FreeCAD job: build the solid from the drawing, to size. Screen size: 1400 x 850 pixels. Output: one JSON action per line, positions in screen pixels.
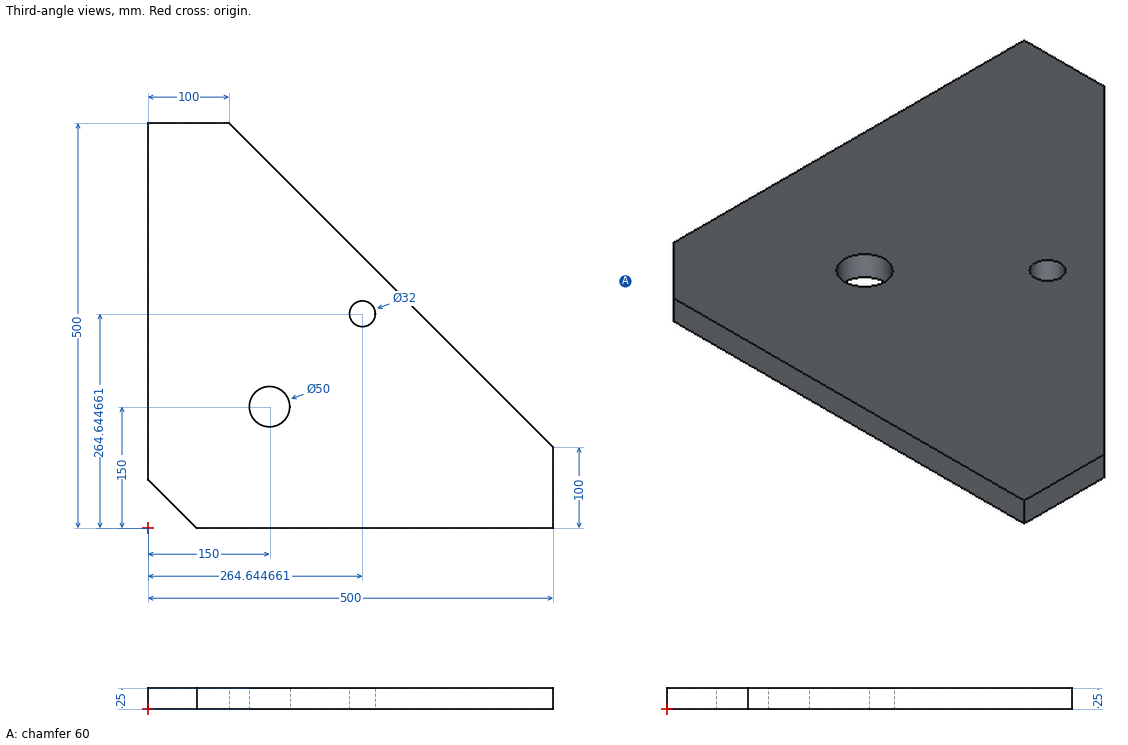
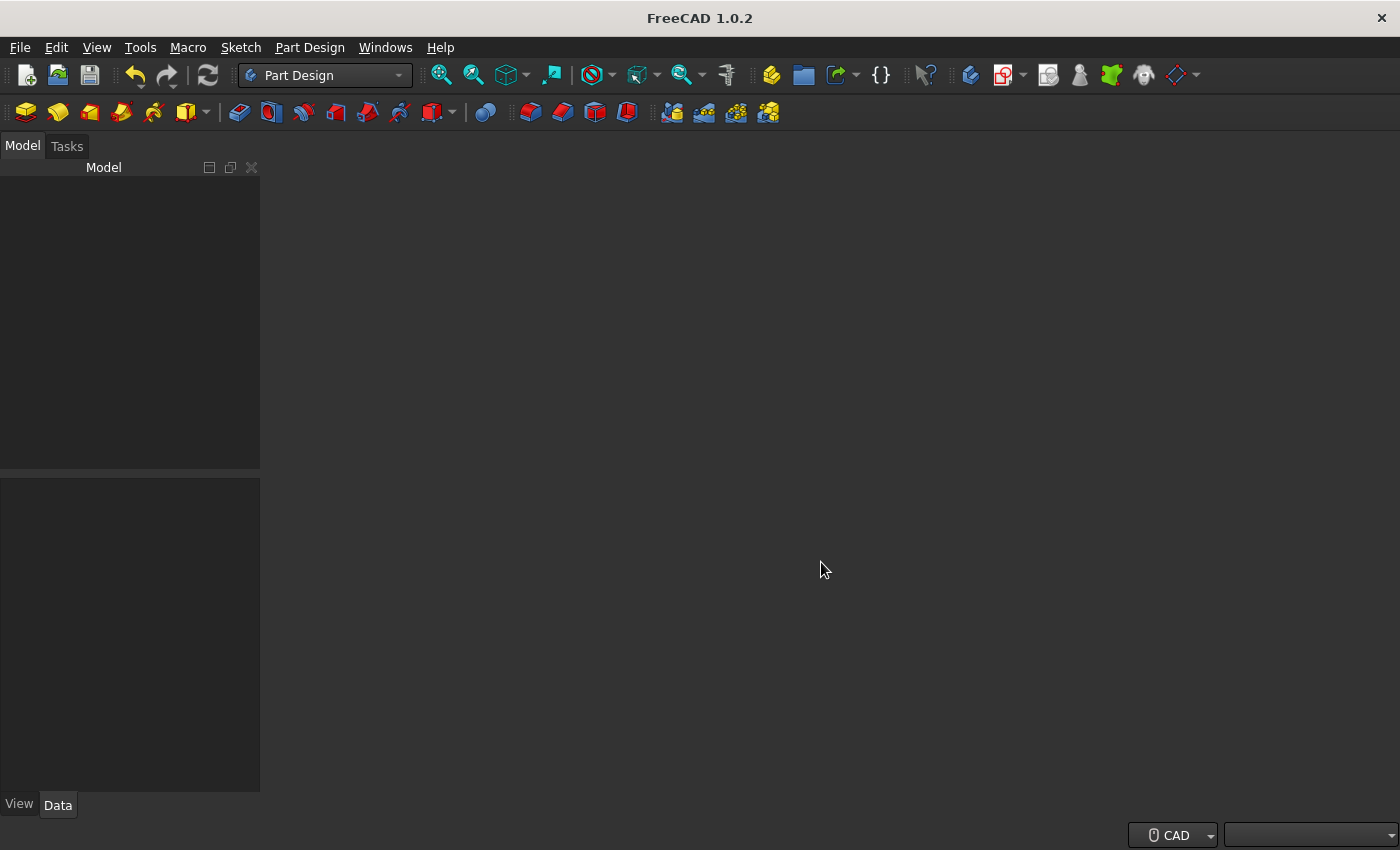
{"action": "left_click", "coordinate": [26, 76]}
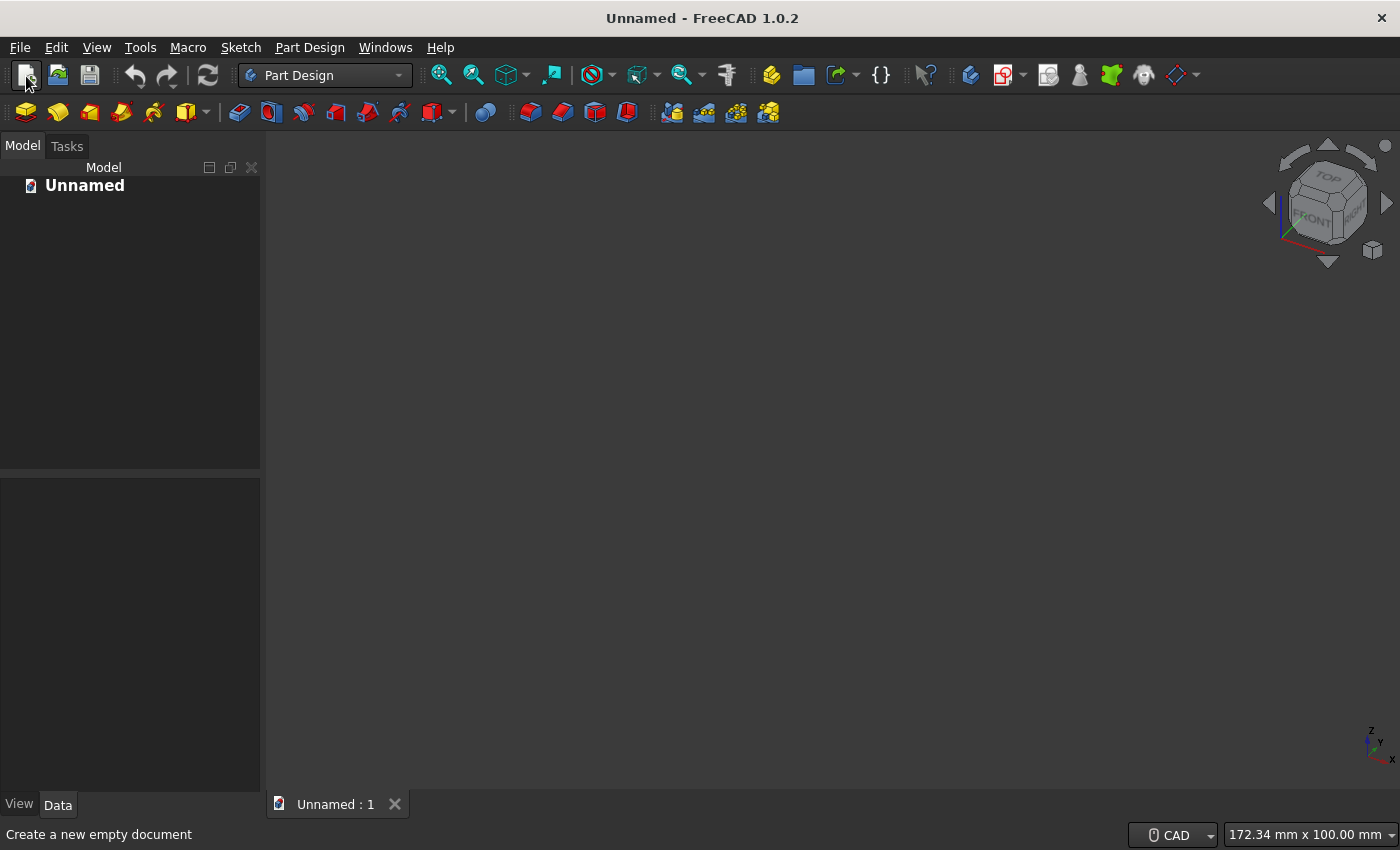
{"action": "left_click", "coordinate": [1004, 76]}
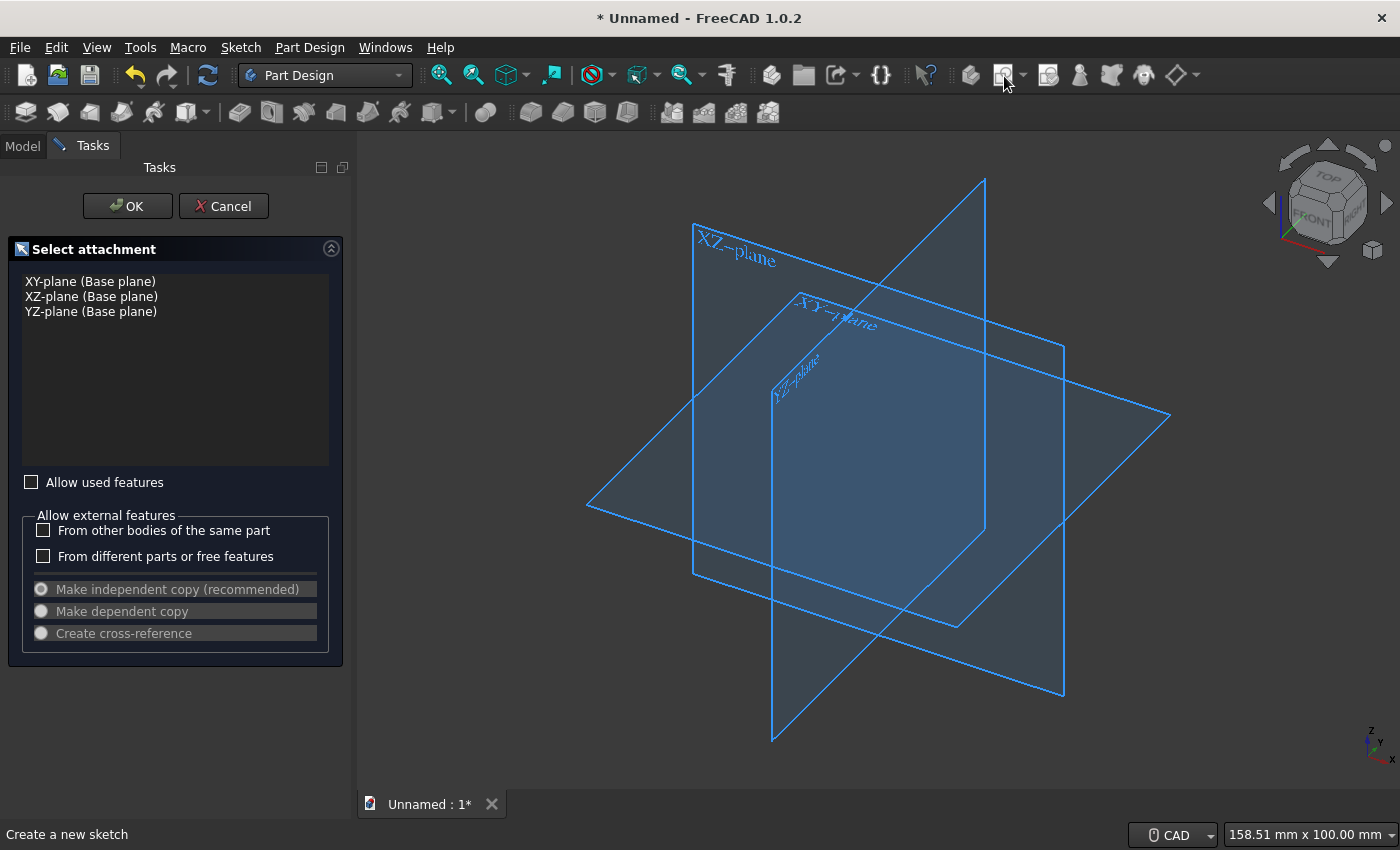
{"action": "left_click", "coordinate": [82, 282]}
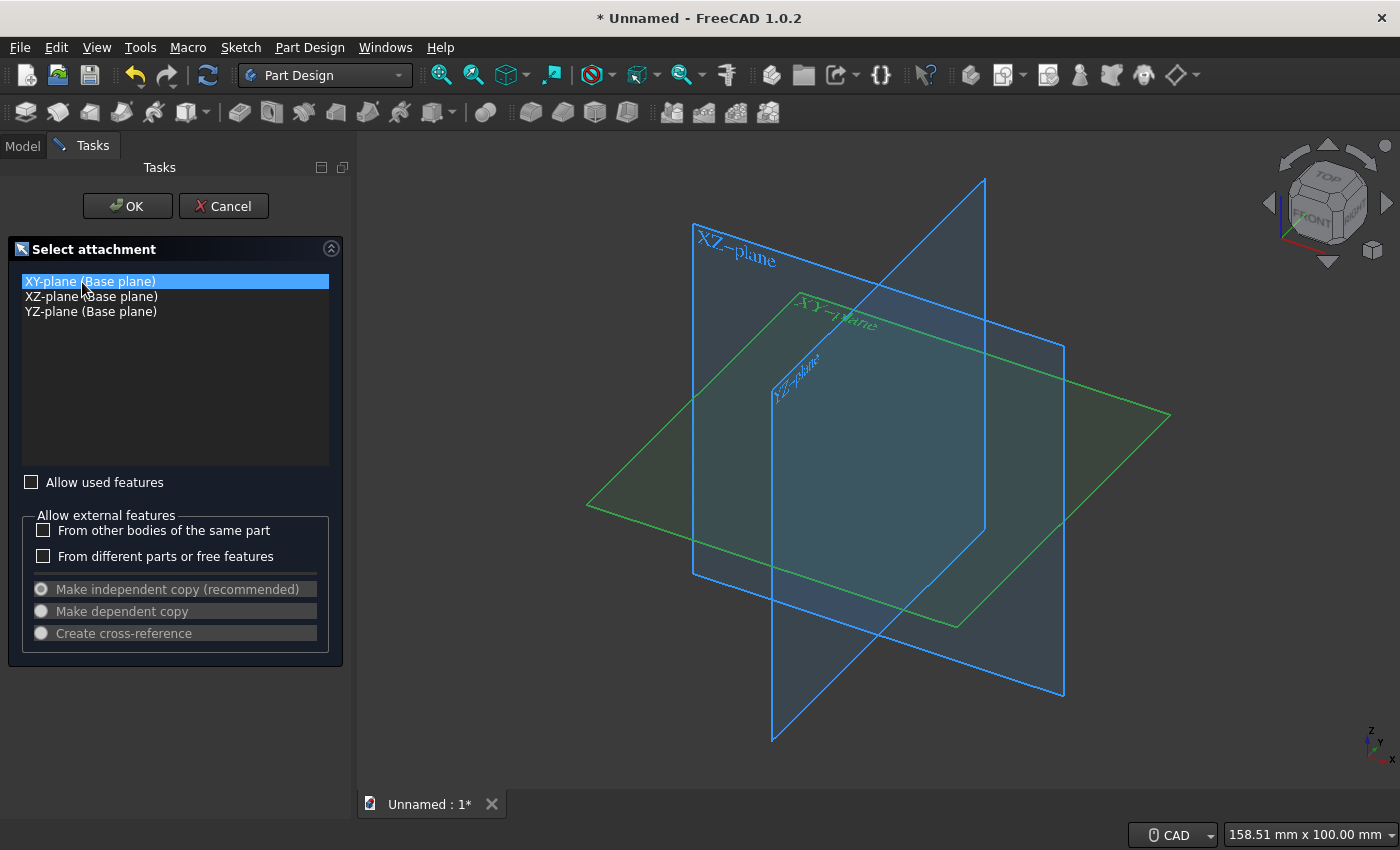
{"action": "left_click", "coordinate": [128, 206]}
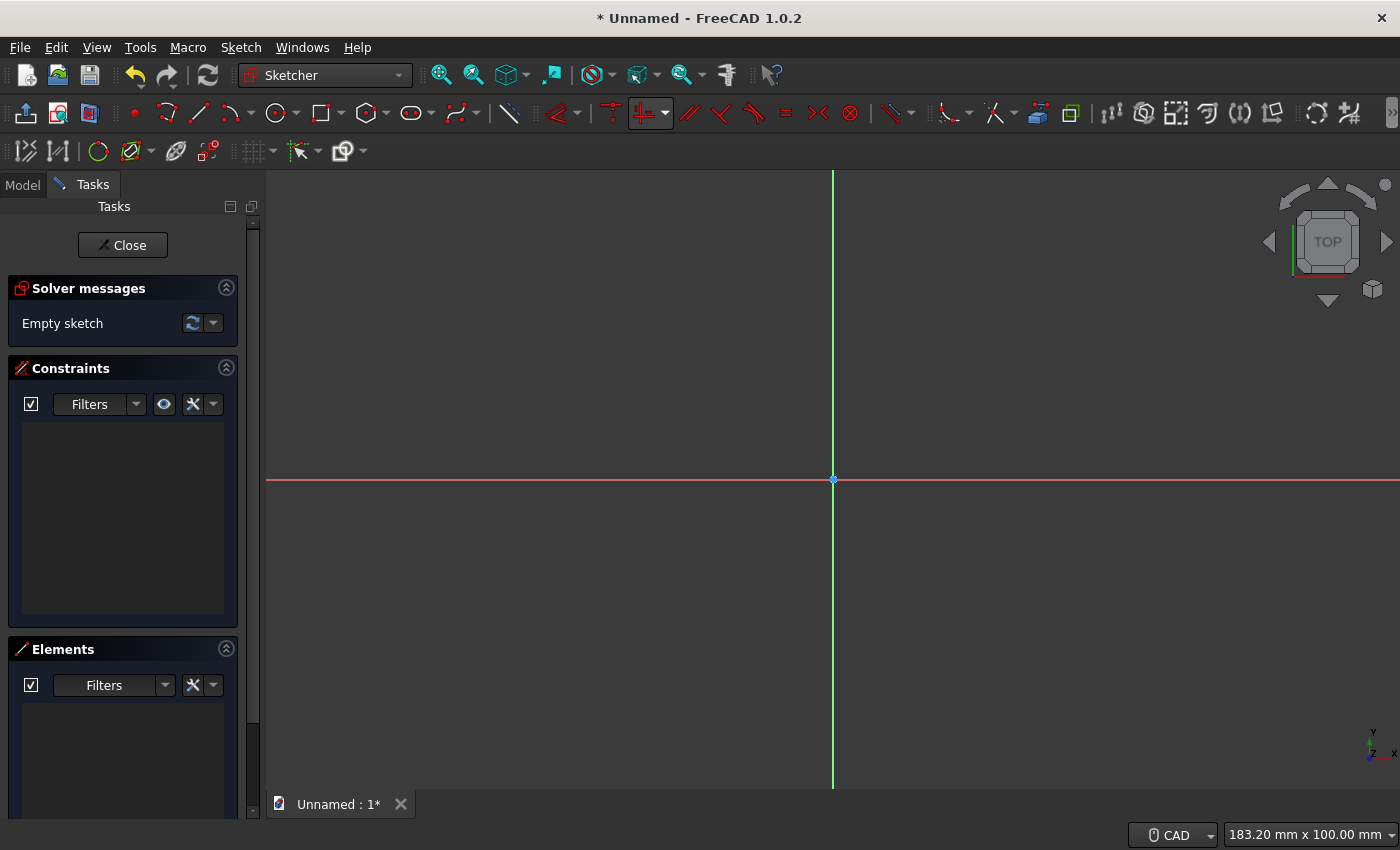
{"action": "scroll", "coordinate": [512, 722], "scroll_direction": "down", "scroll_amount": 10}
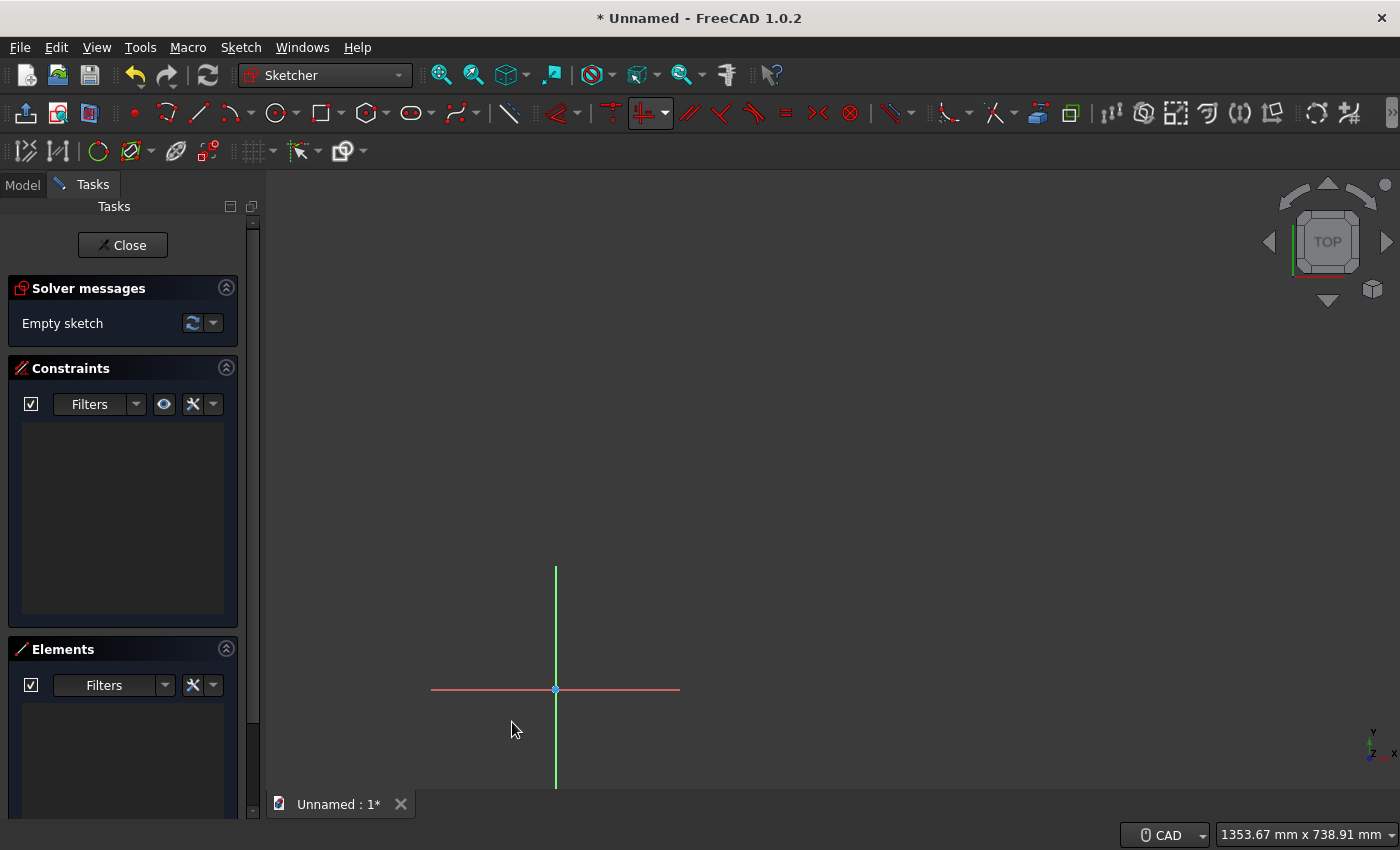
{"action": "left_click", "coordinate": [168, 114]}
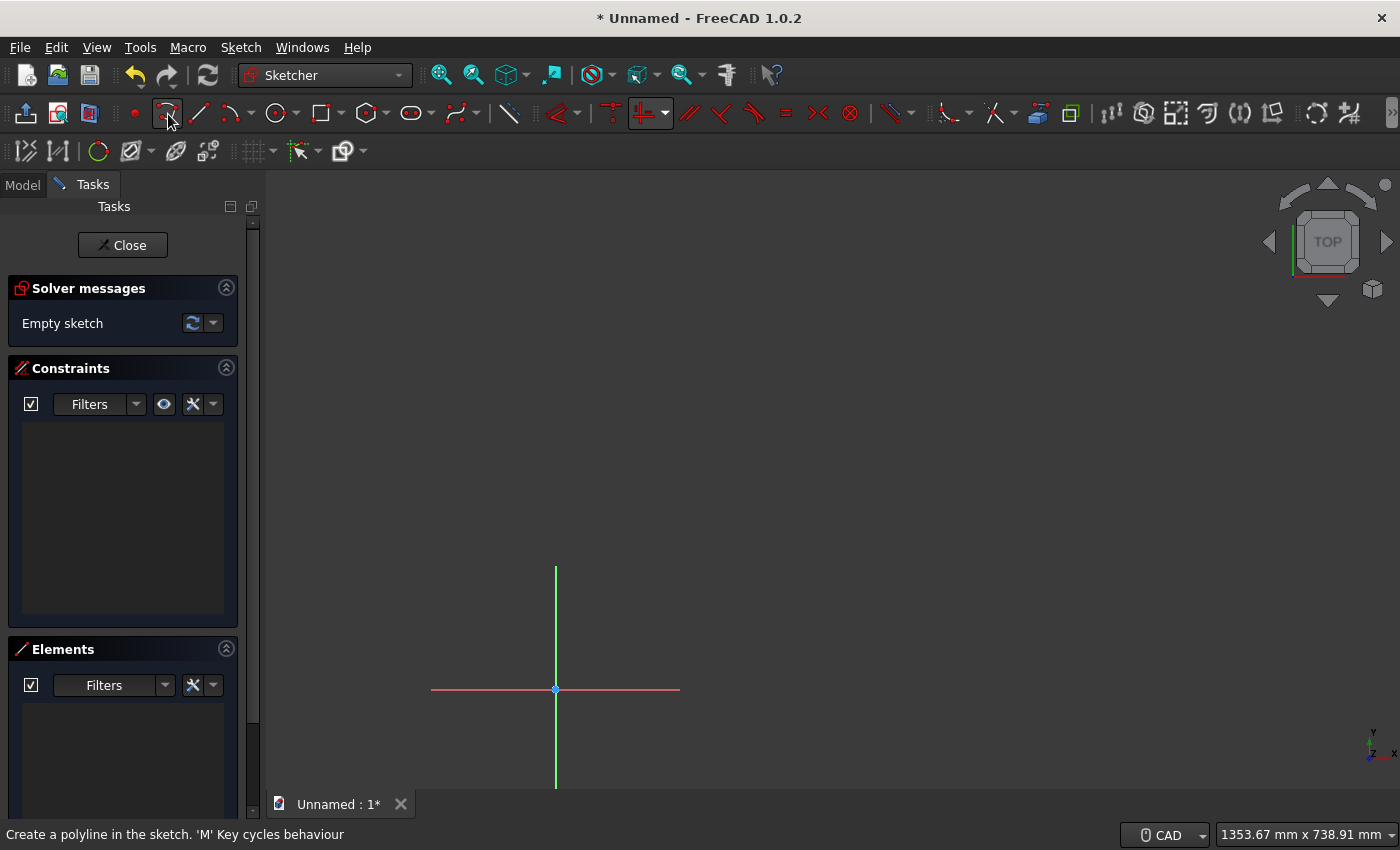
{"action": "left_click", "coordinate": [556, 690]}
{"action": "left_click", "coordinate": [974, 681]}
{"action": "left_click", "coordinate": [974, 606]}
{"action": "left_click", "coordinate": [639, 271]}
{"action": "left_click", "coordinate": [565, 271]}
{"action": "left_click", "coordinate": [556, 690]}
{"action": "key", "text": "Escape"}
{"action": "key", "text": "Escape"}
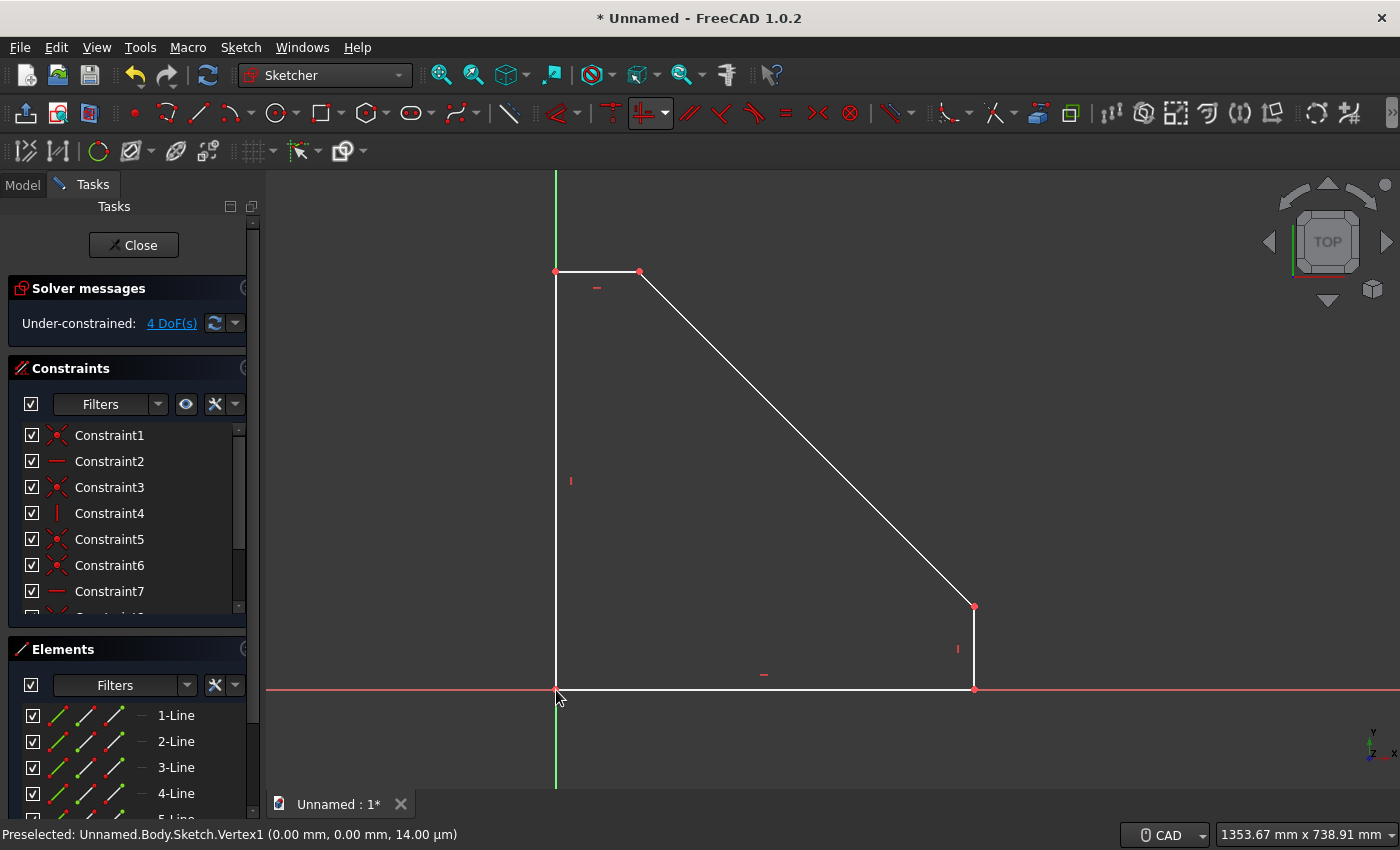
{"action": "left_click", "coordinate": [556, 114]}